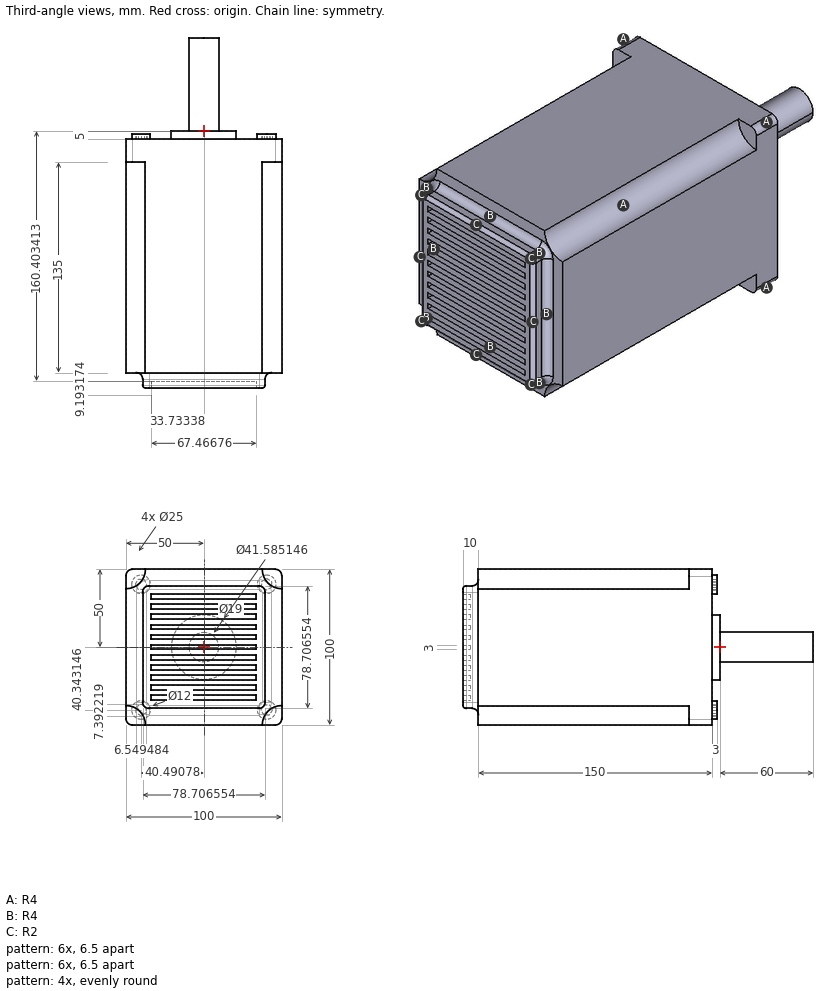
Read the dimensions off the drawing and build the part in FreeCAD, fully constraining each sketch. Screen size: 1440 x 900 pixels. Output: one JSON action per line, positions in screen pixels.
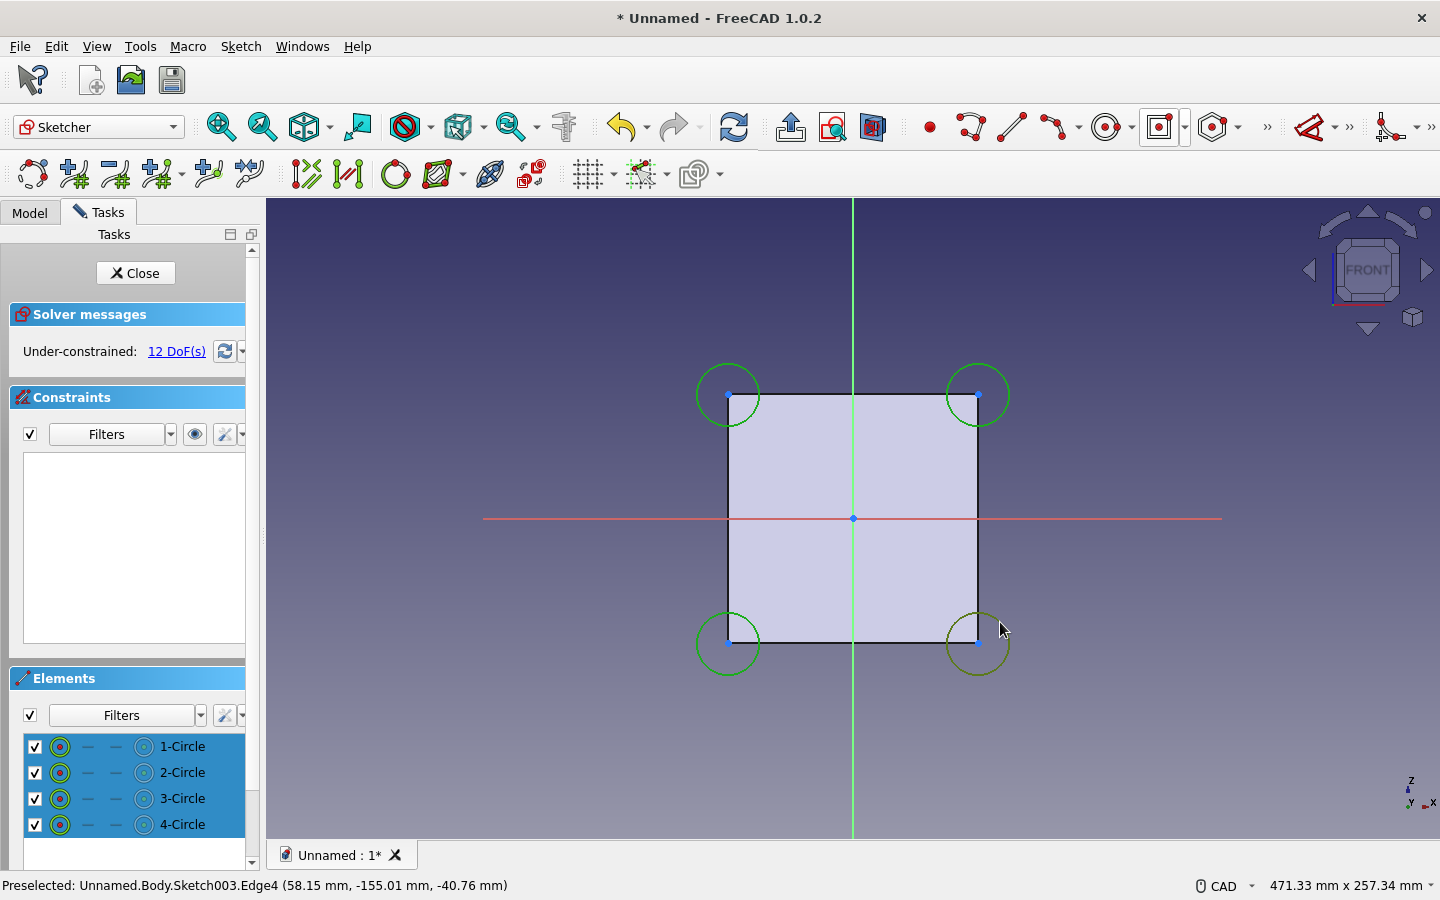
{"action": "key", "text": "e"}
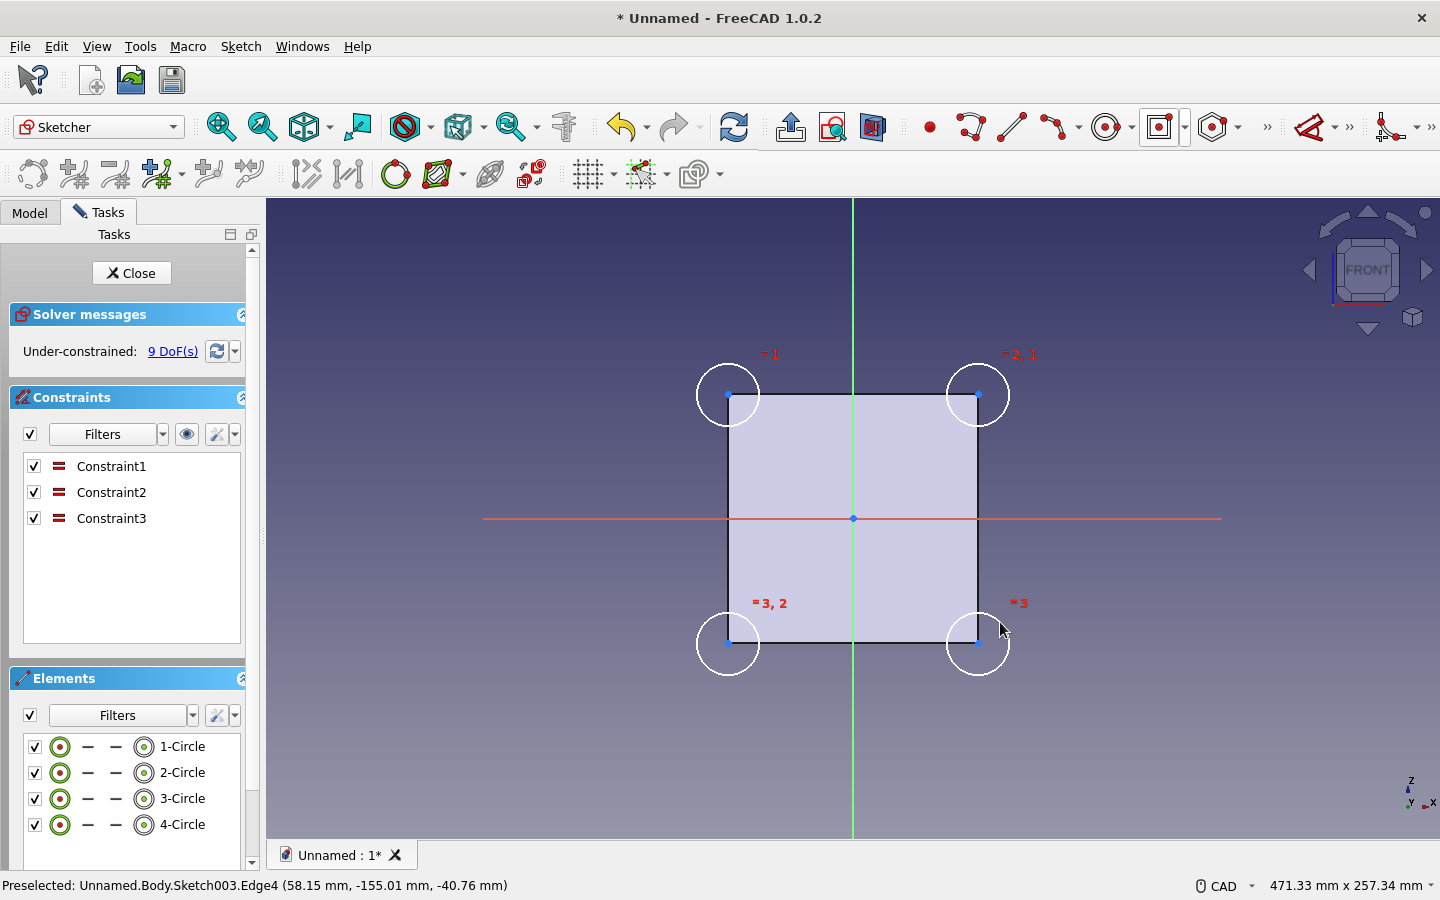
{"action": "left_click", "coordinate": [728, 395]}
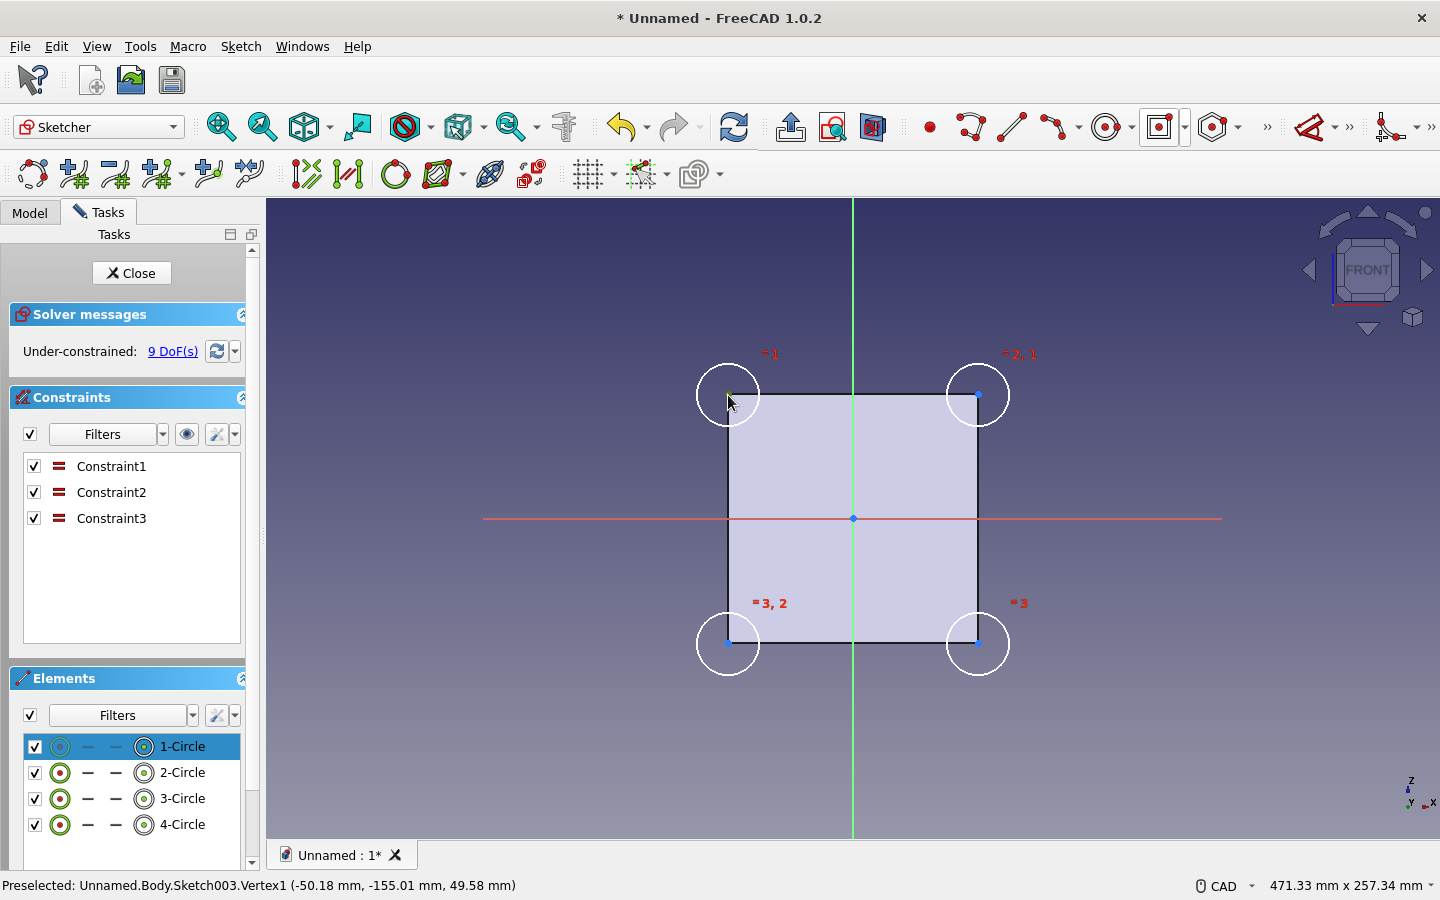
{"action": "left_click", "coordinate": [978, 395]}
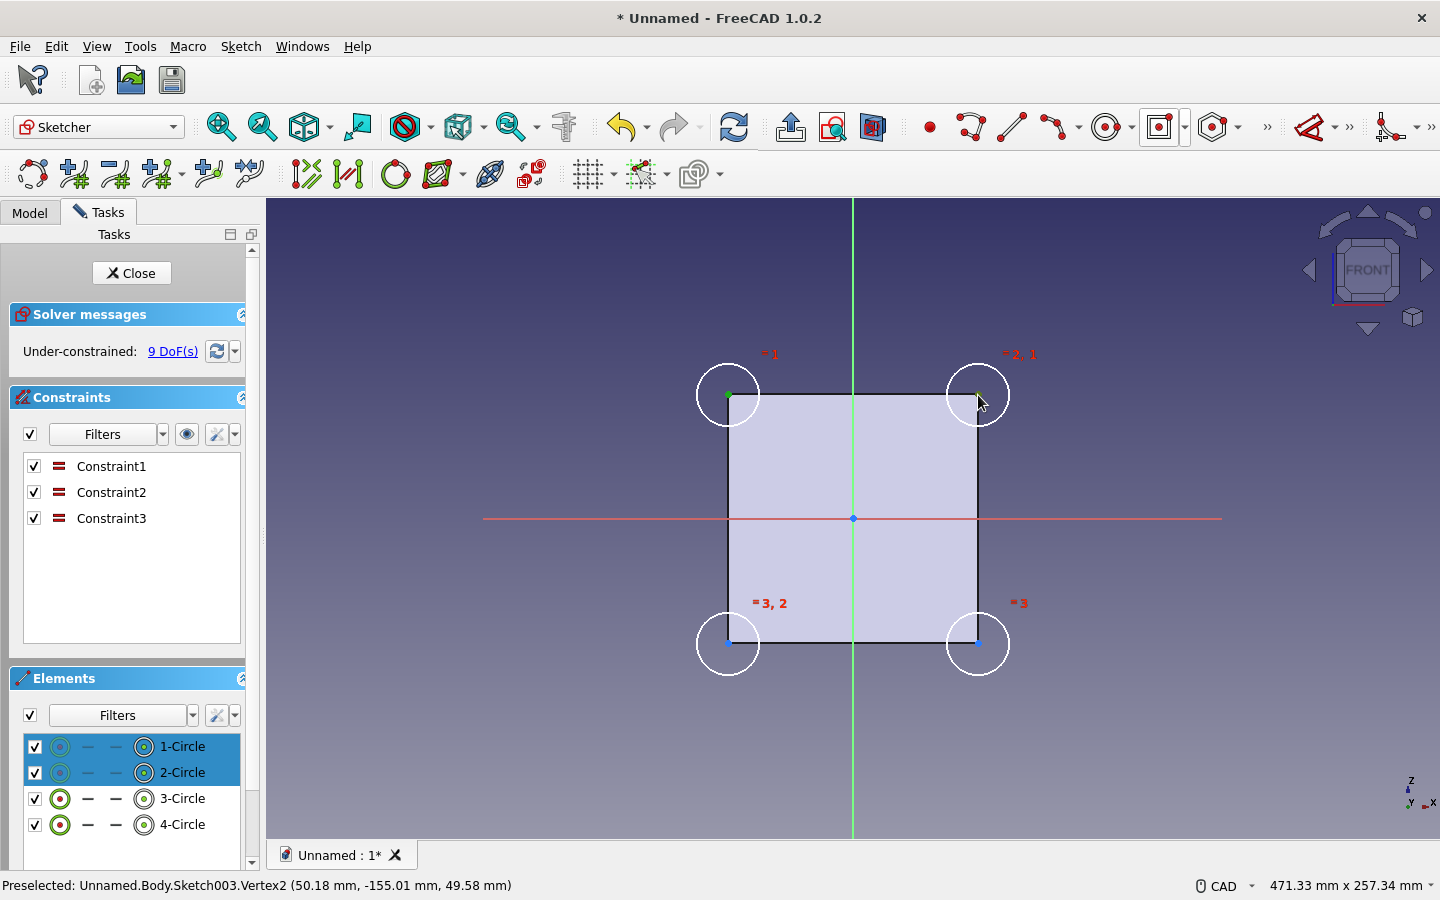
{"action": "left_click", "coordinate": [853, 769]}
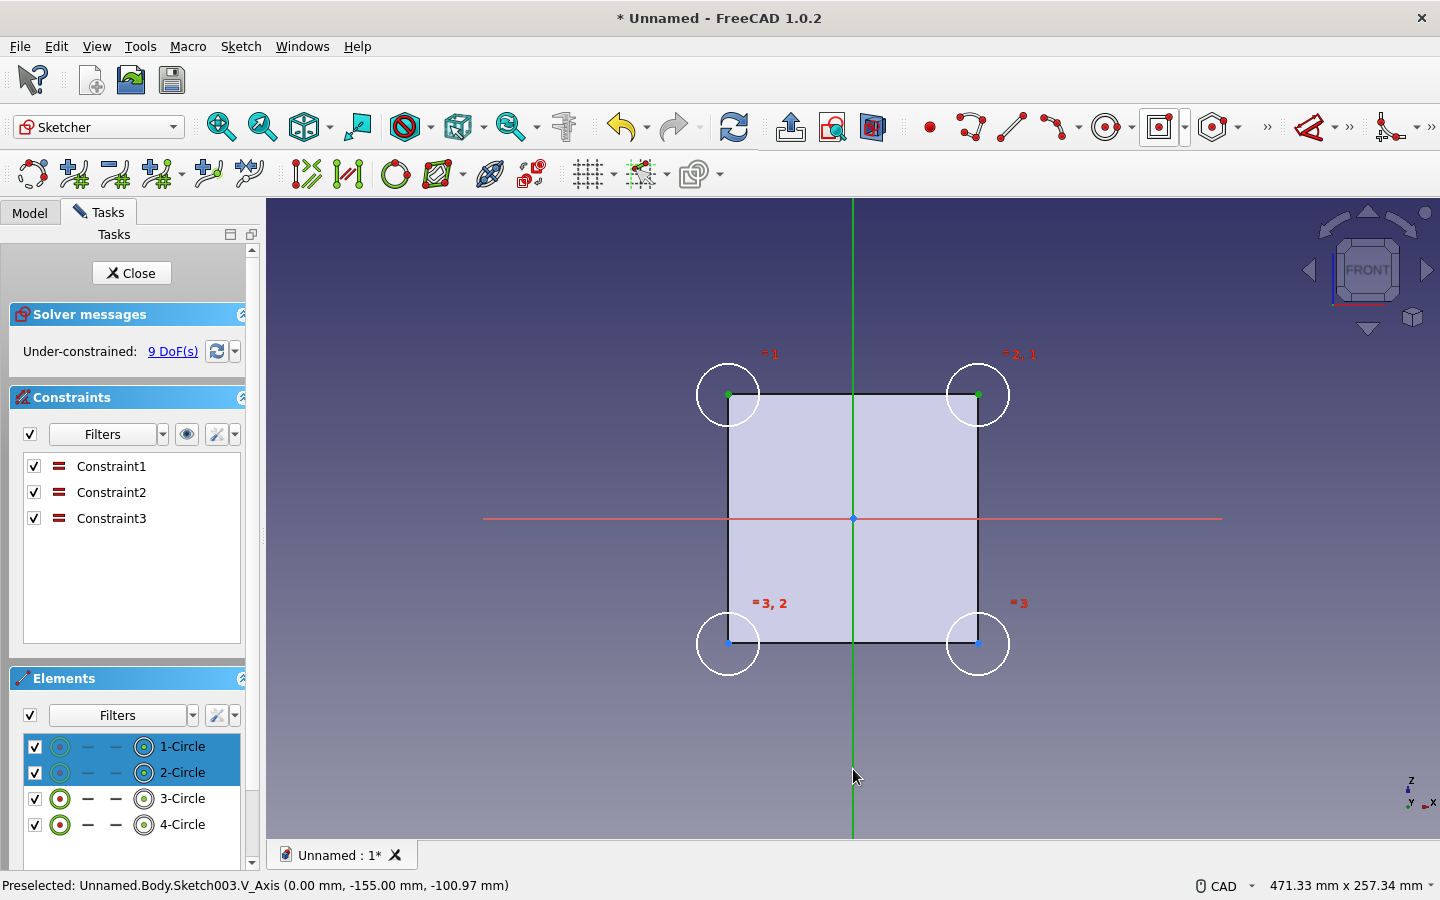
{"action": "key", "text": "s"}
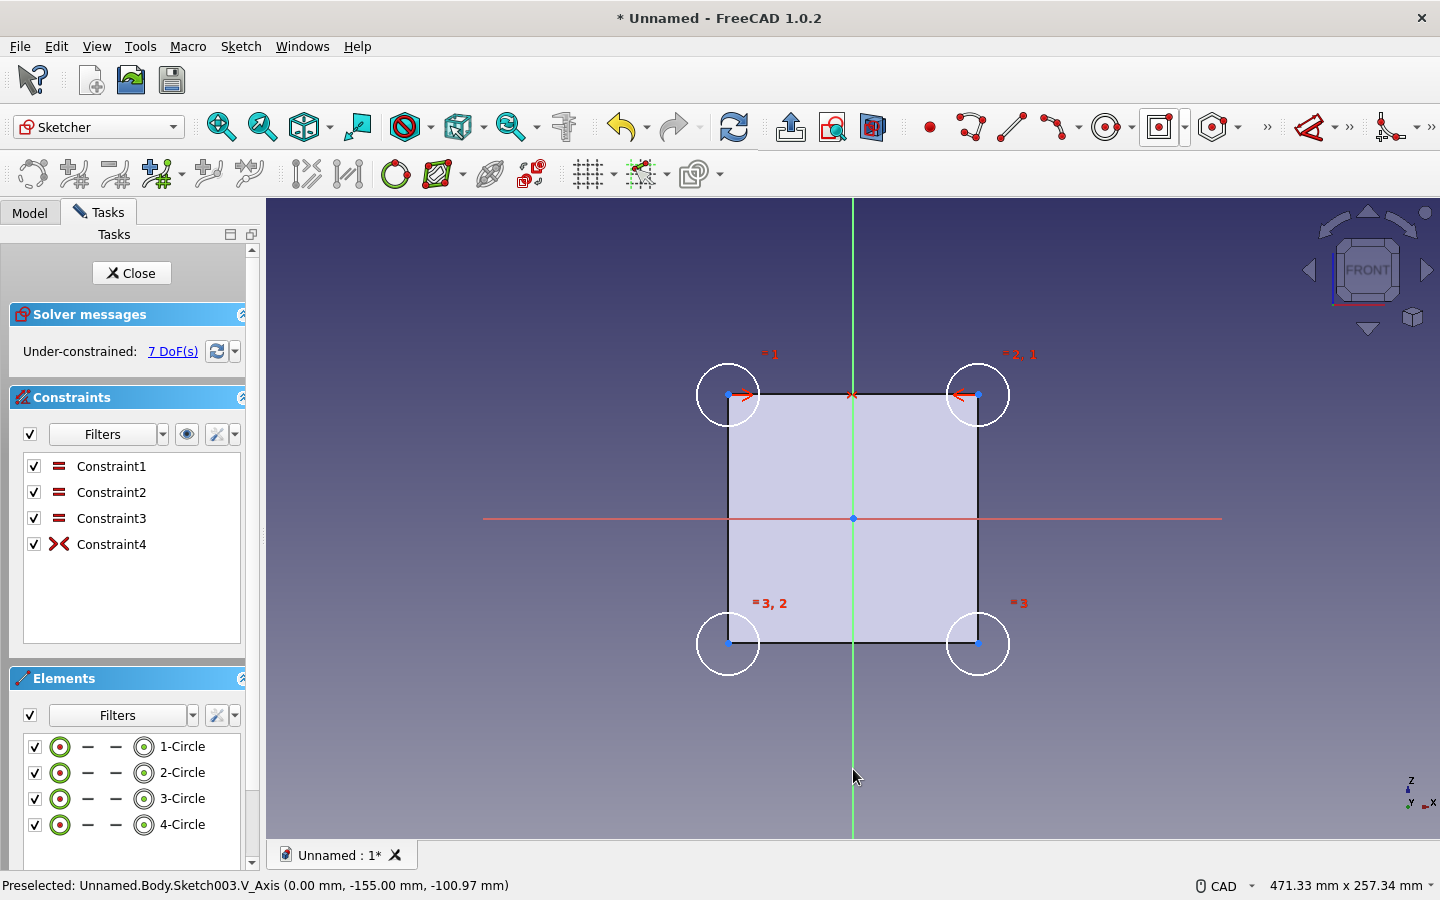
{"action": "left_click", "coordinate": [728, 395]}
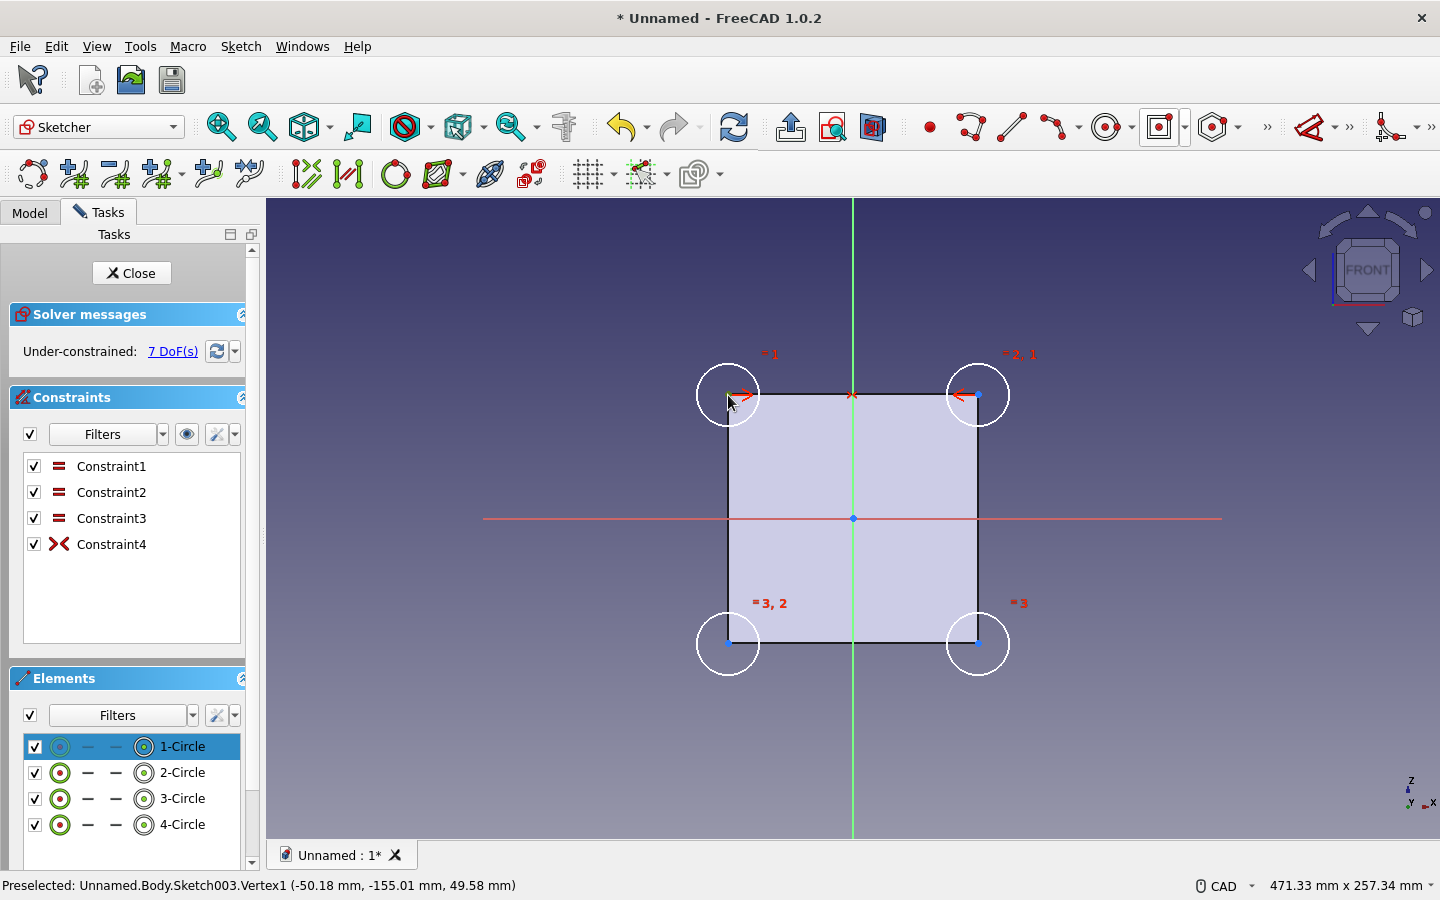
{"action": "left_click", "coordinate": [728, 644]}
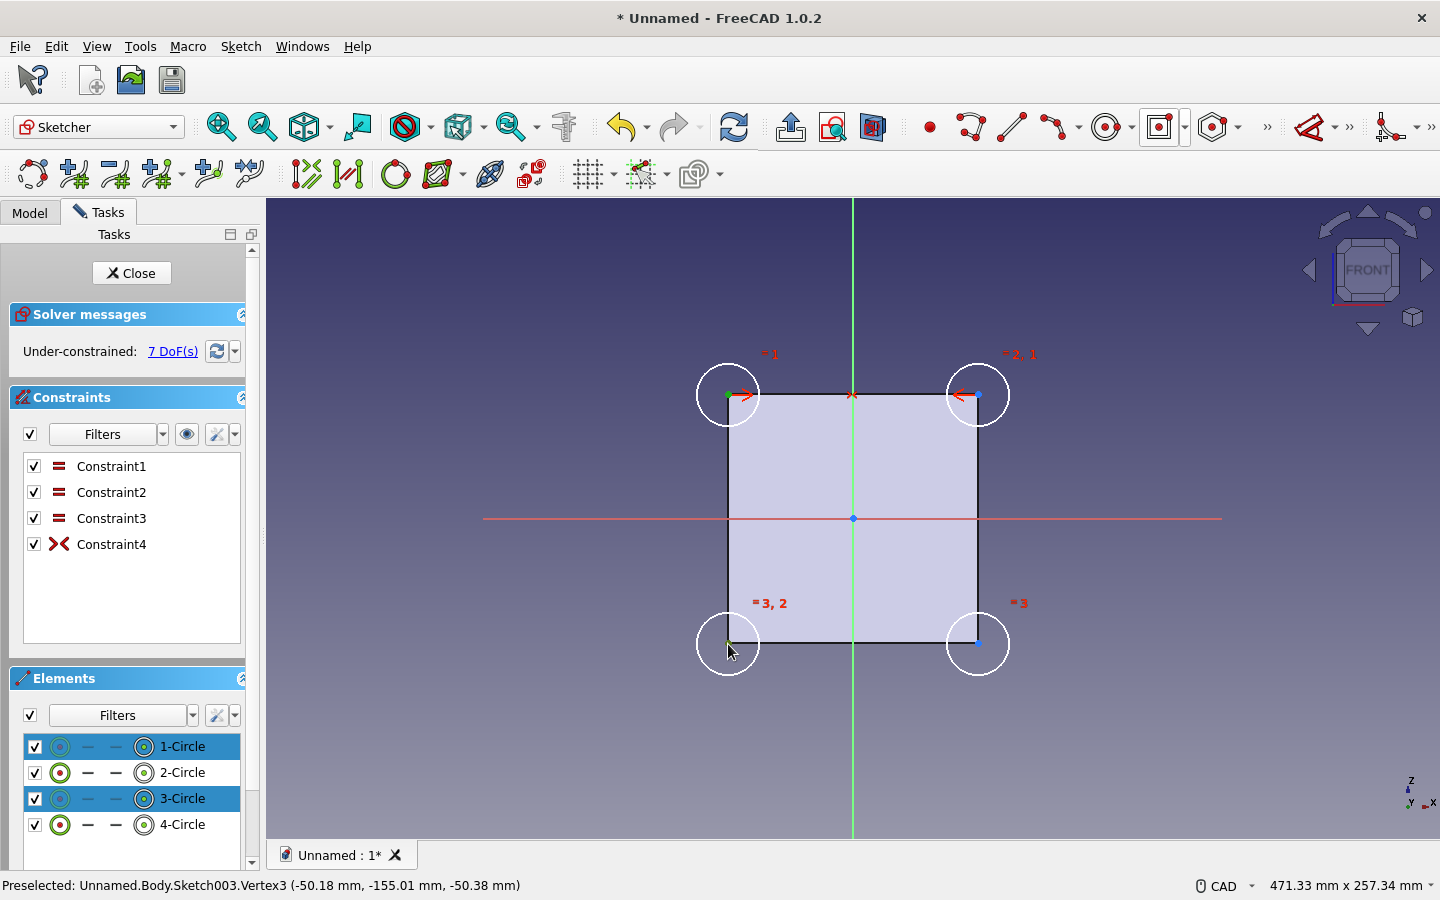
{"action": "left_click", "coordinate": [504, 518]}